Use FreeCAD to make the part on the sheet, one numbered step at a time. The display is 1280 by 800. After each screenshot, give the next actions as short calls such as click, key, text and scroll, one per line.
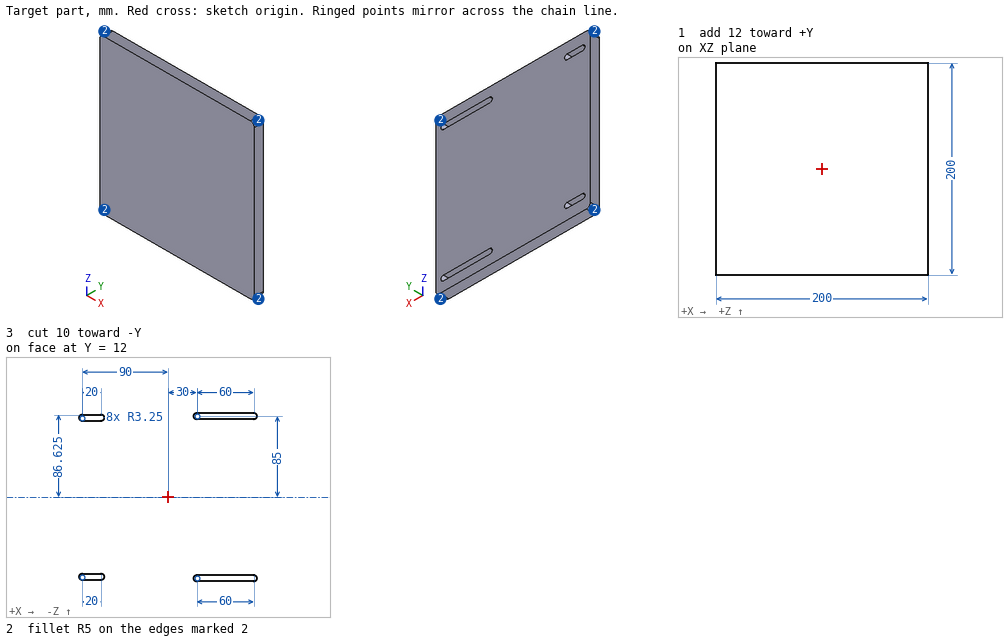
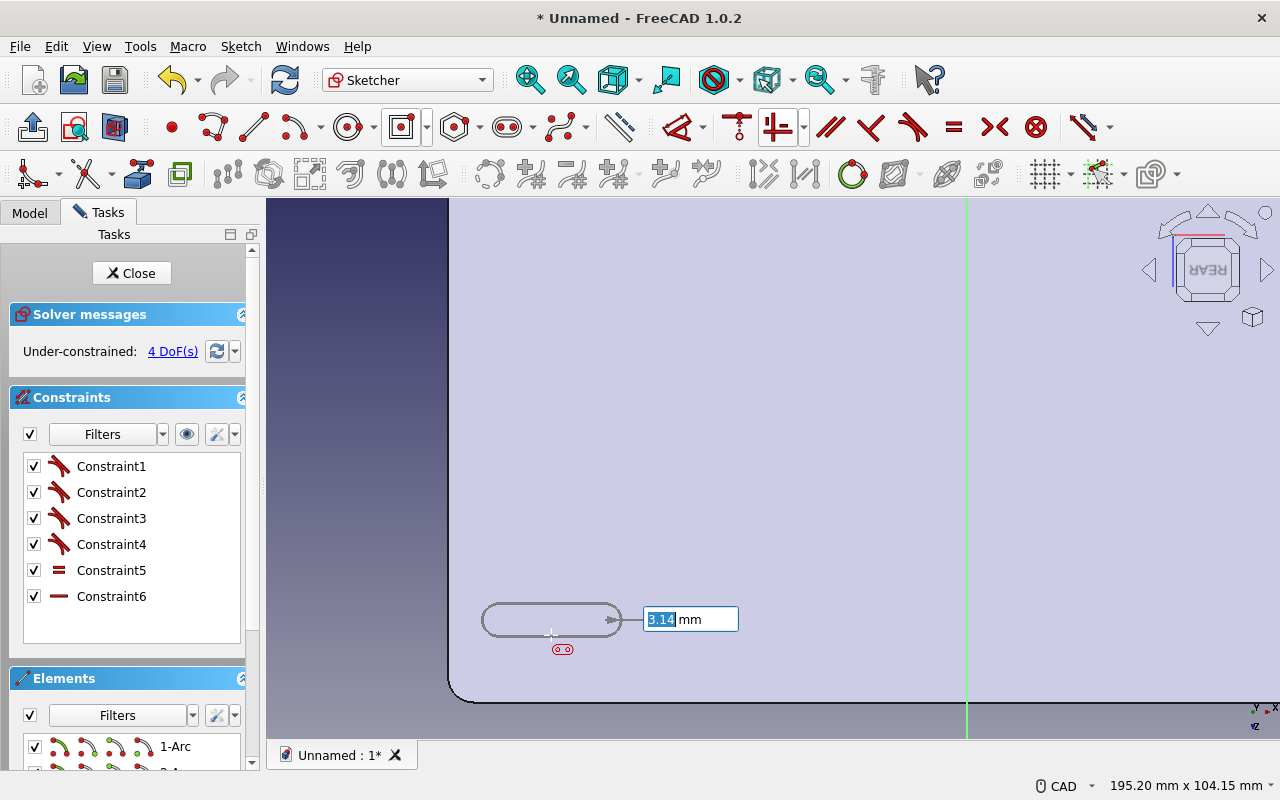
click(552, 633)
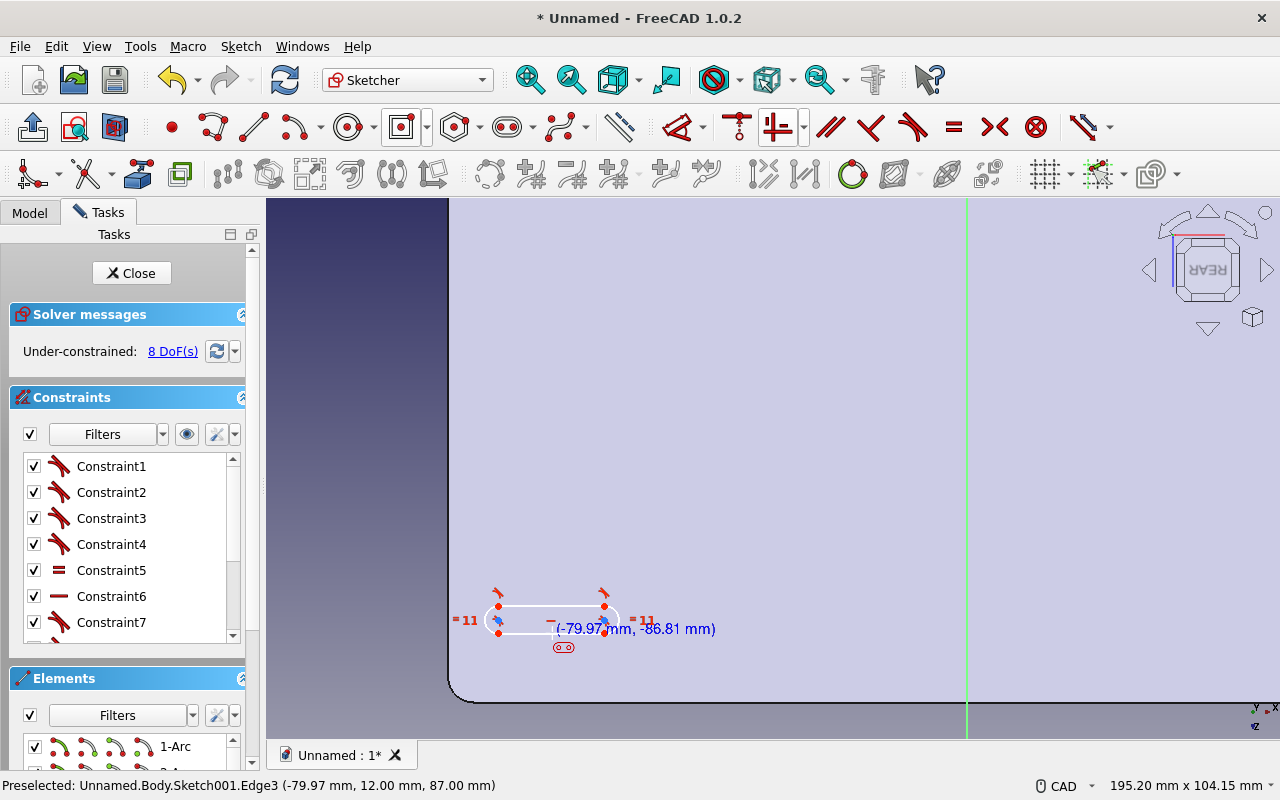
scroll(551, 635, down, 5)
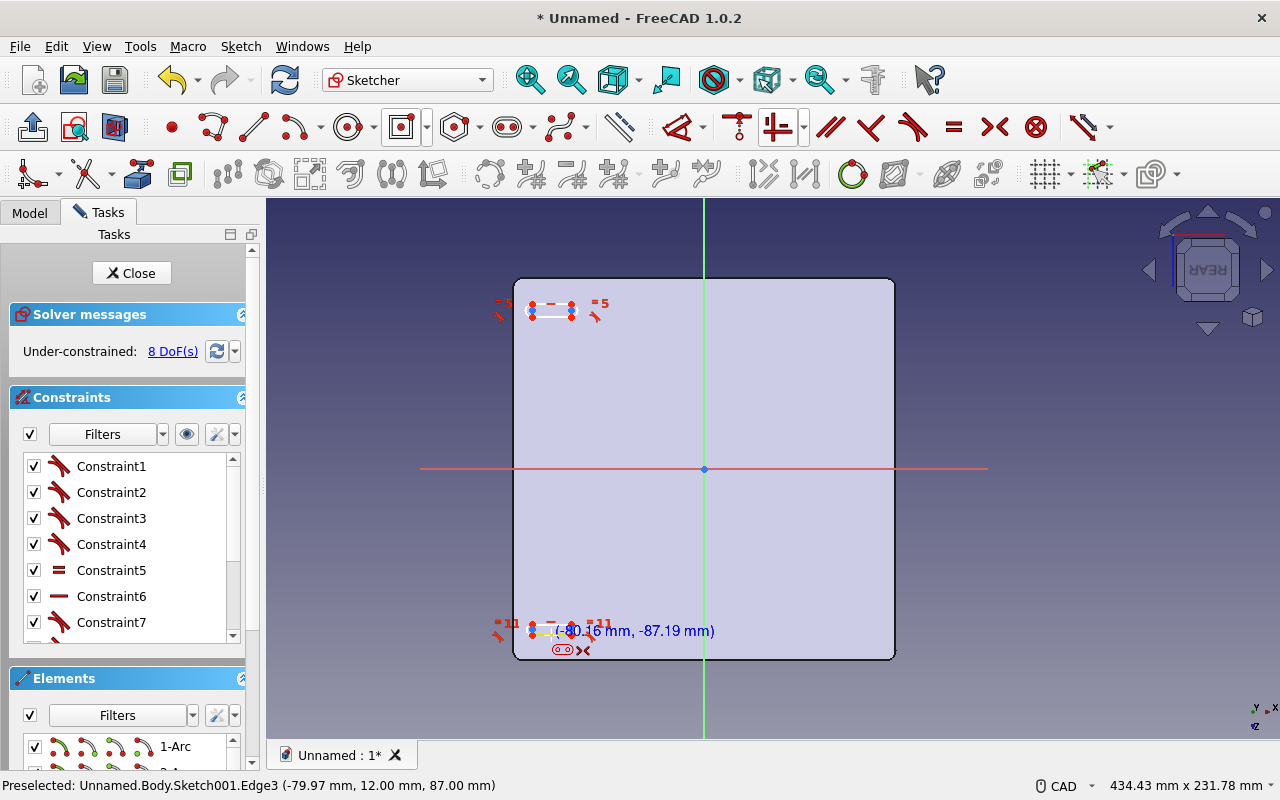
scroll(762, 307, up, 7)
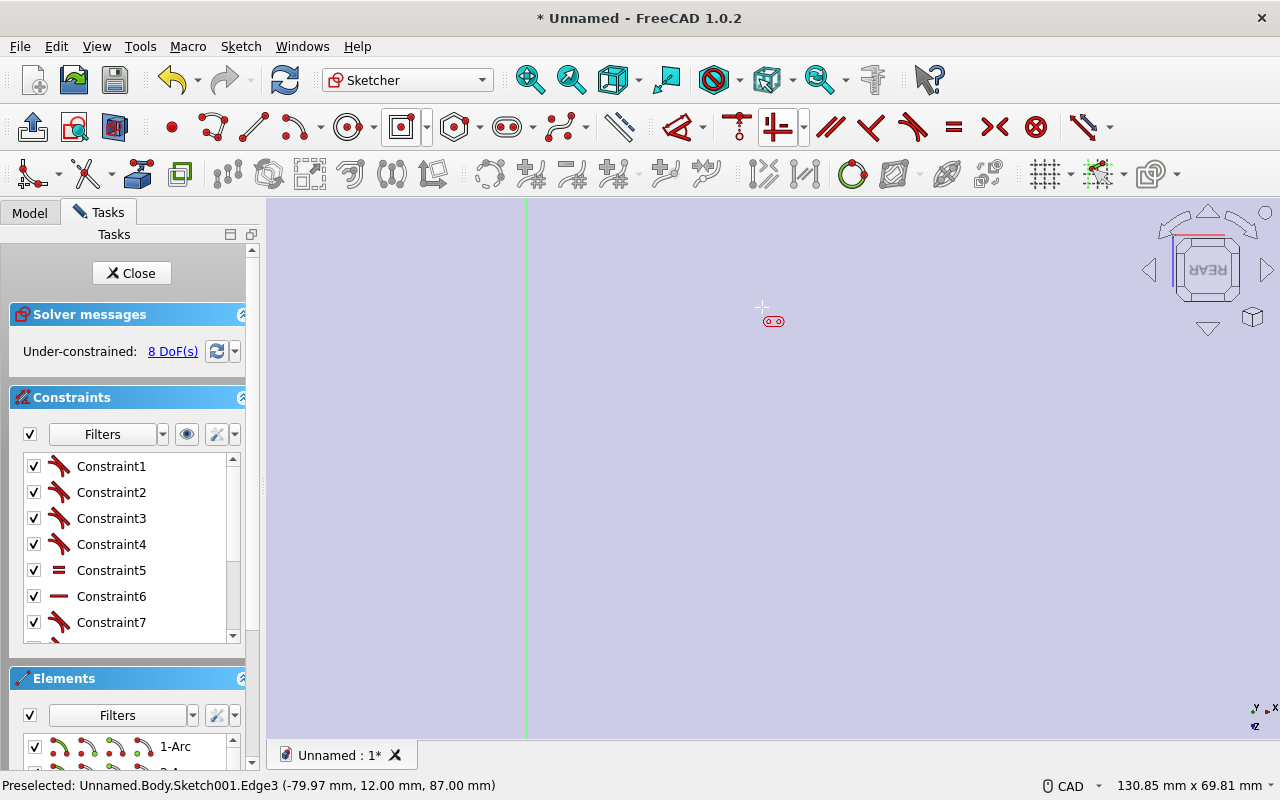
scroll(763, 306, down, 7)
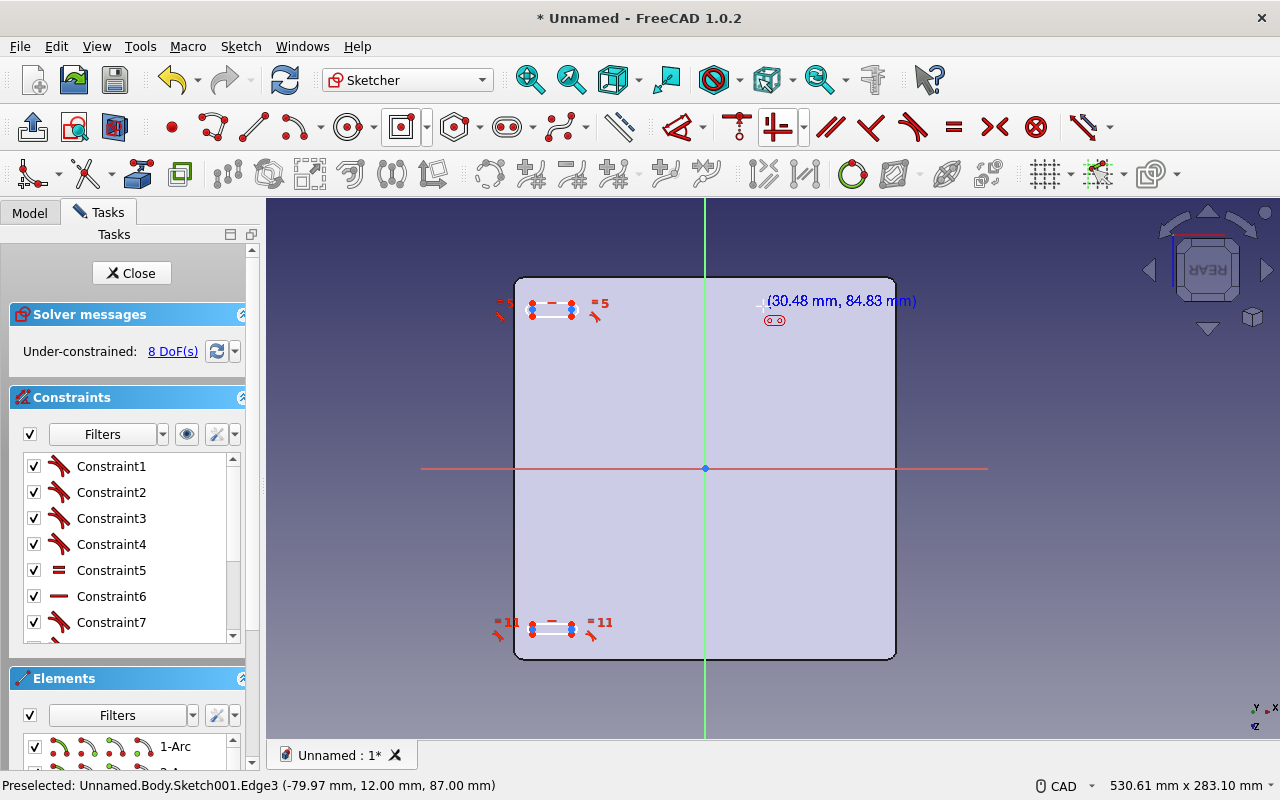
click(762, 306)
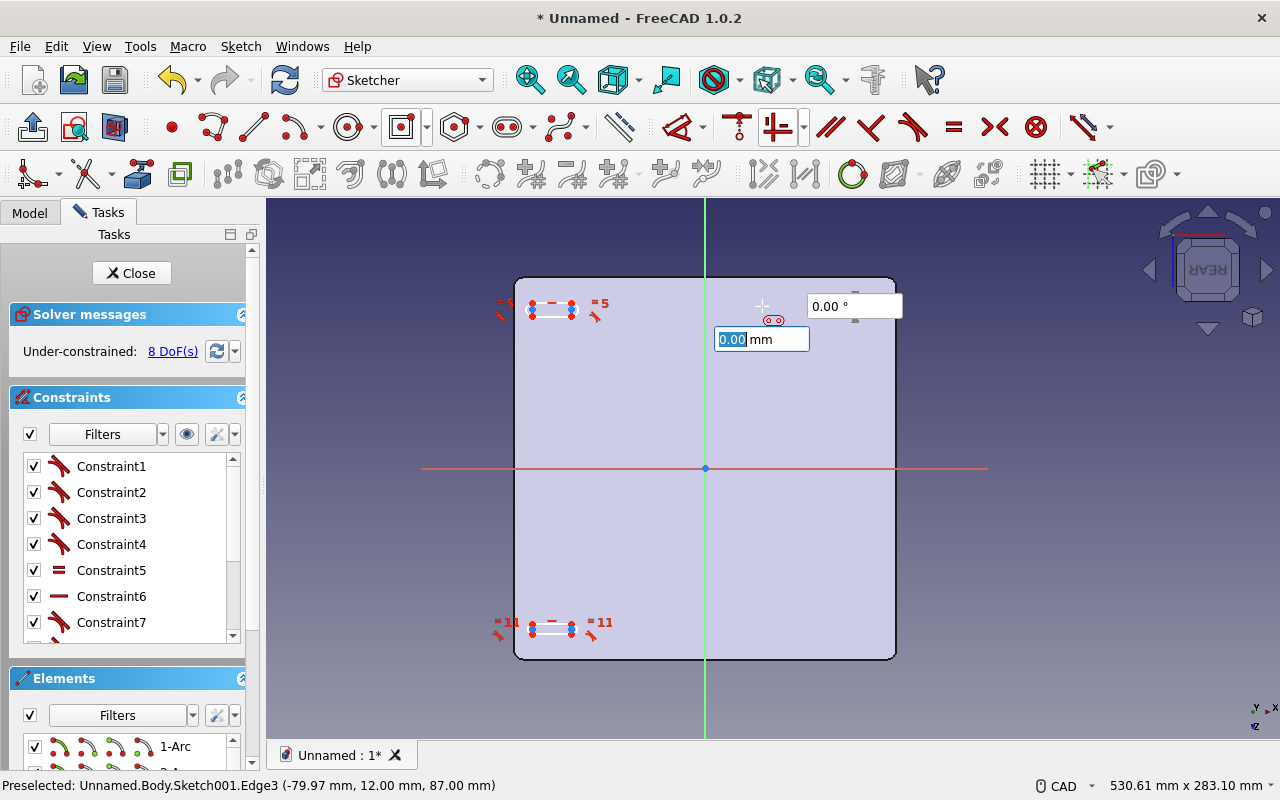
click(877, 306)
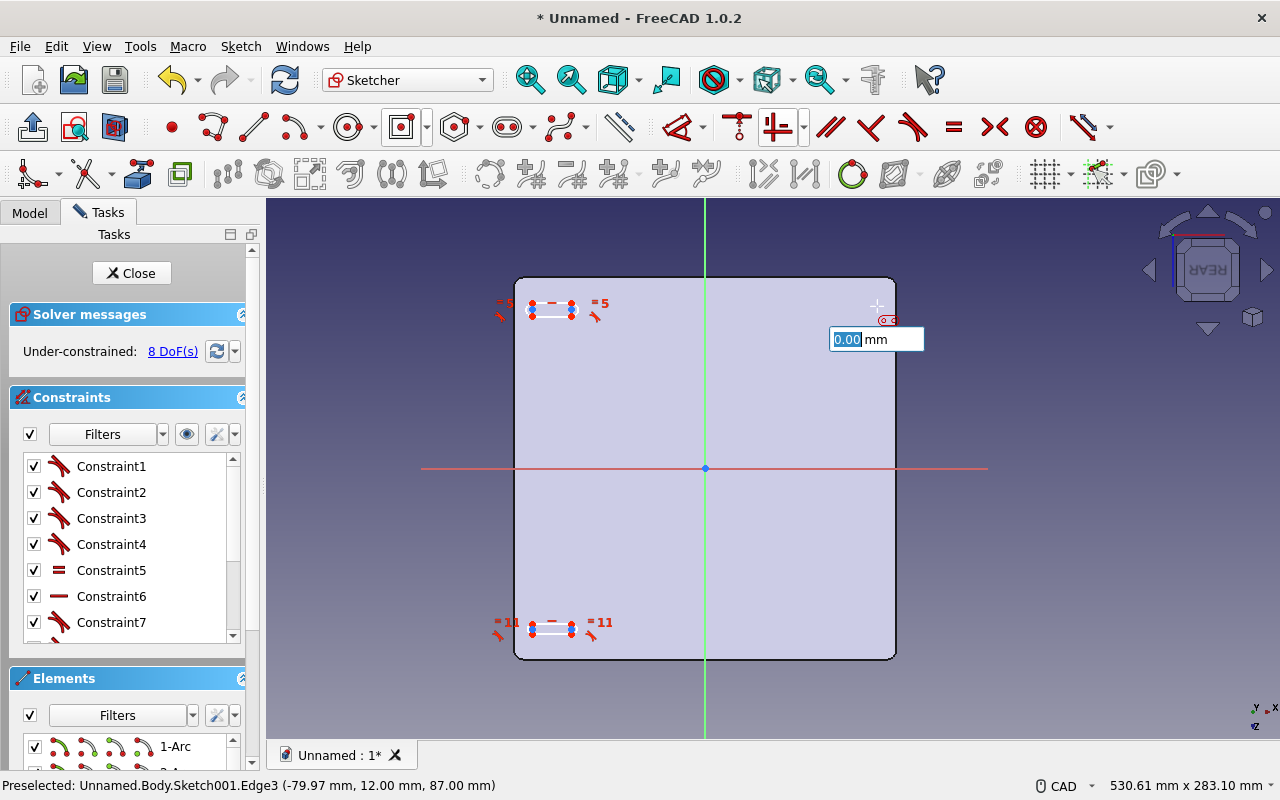
scroll(820, 300, up, 5)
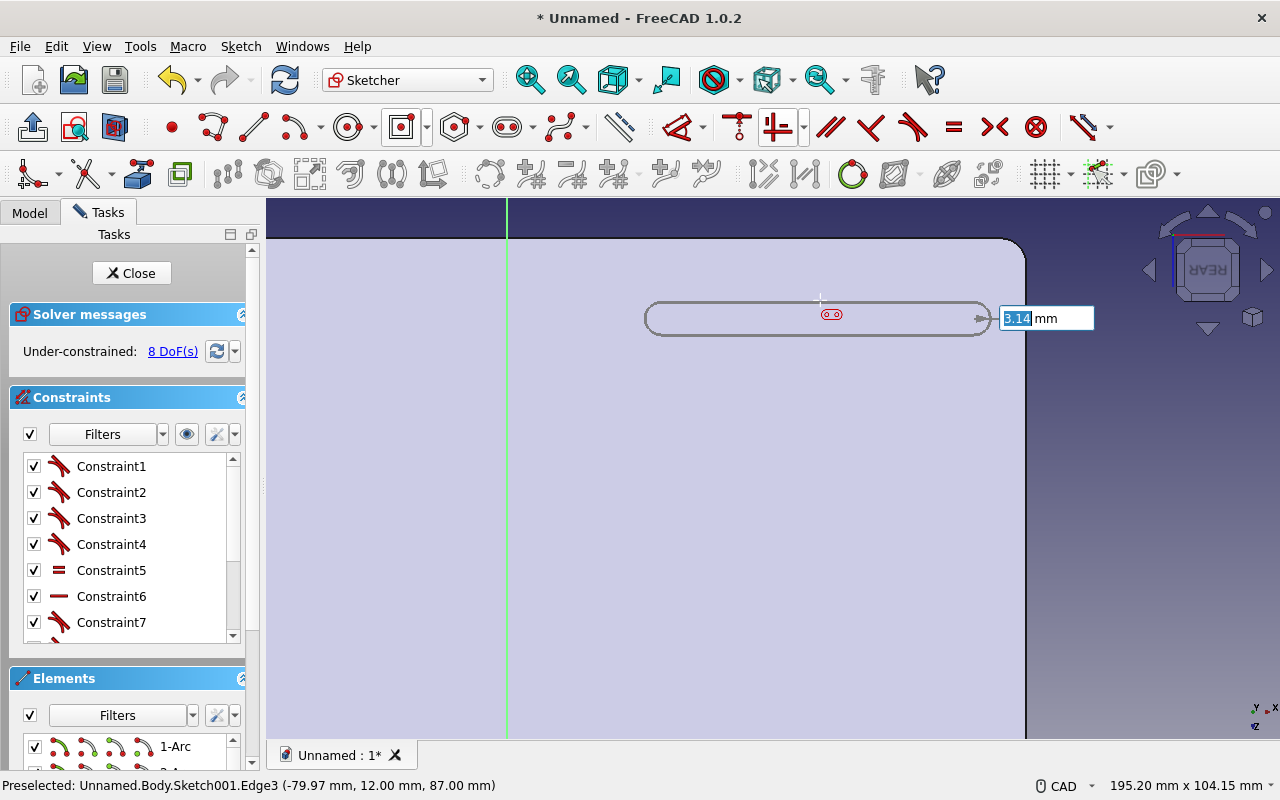
click(818, 299)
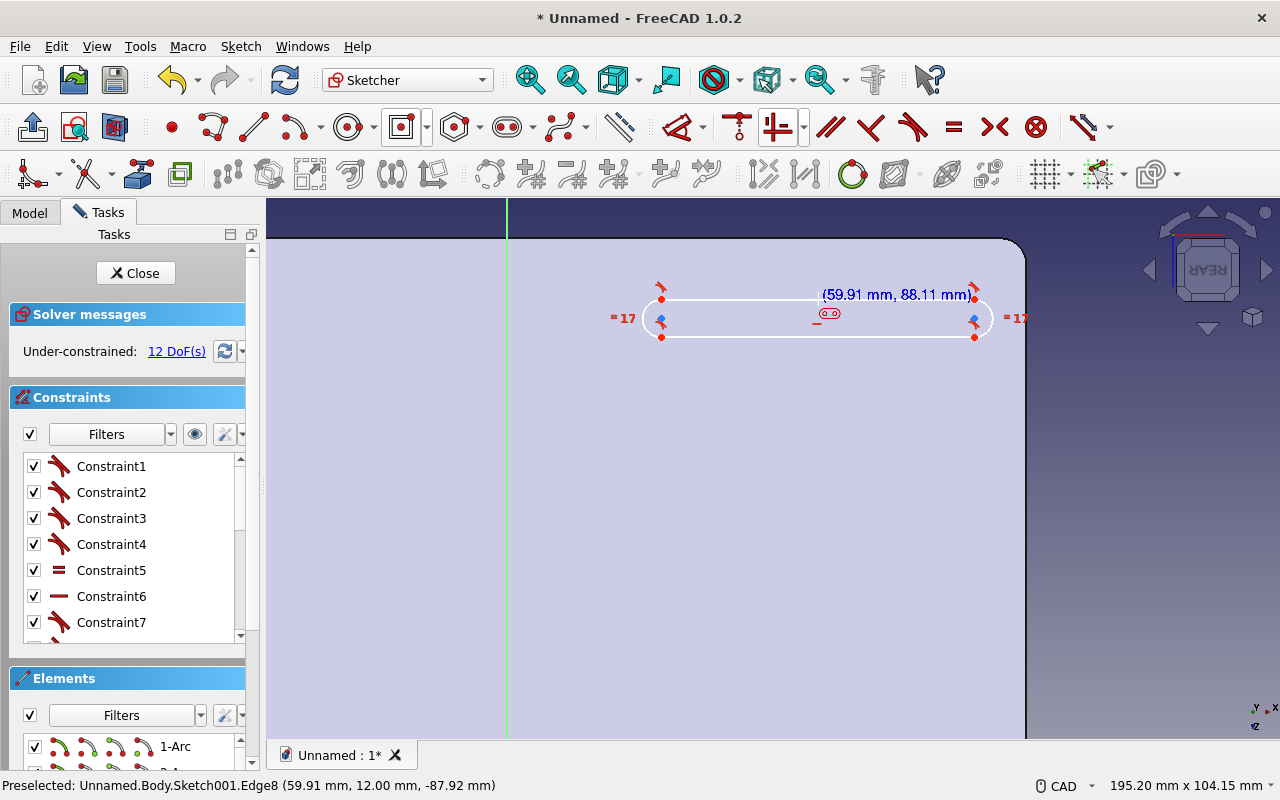
scroll(820, 300, down, 5)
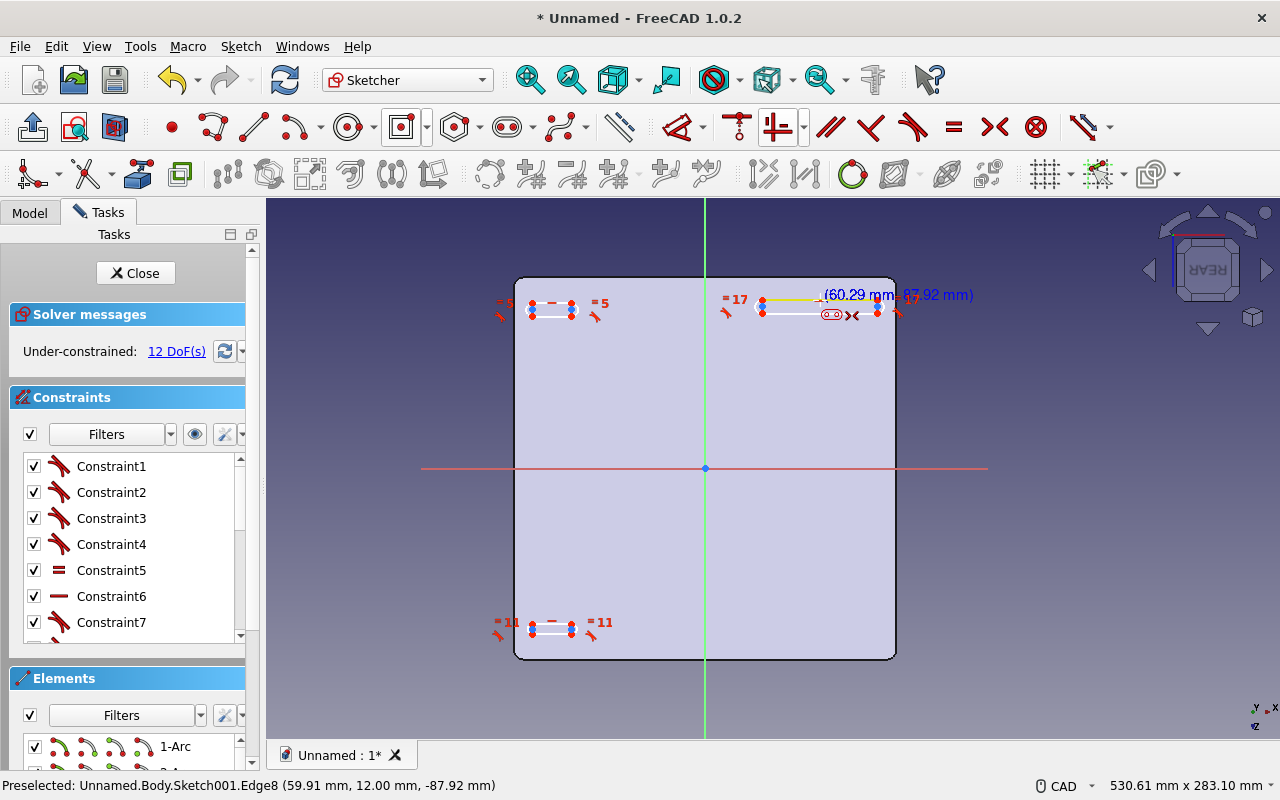
scroll(762, 631, up, 7)